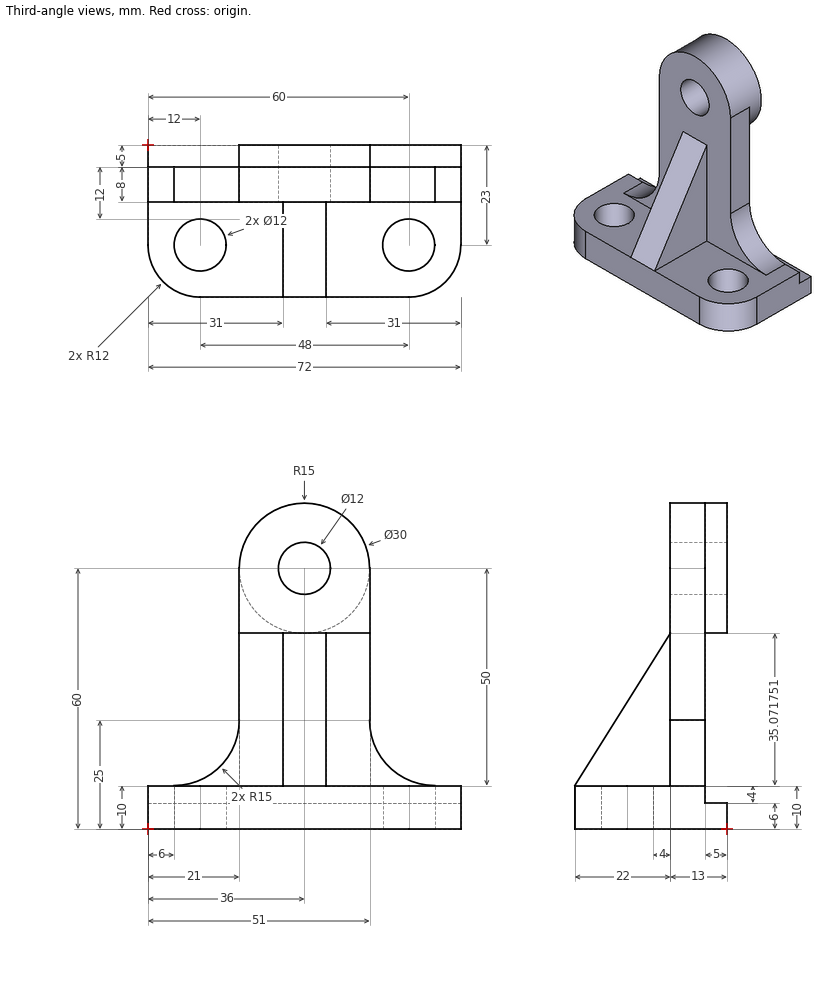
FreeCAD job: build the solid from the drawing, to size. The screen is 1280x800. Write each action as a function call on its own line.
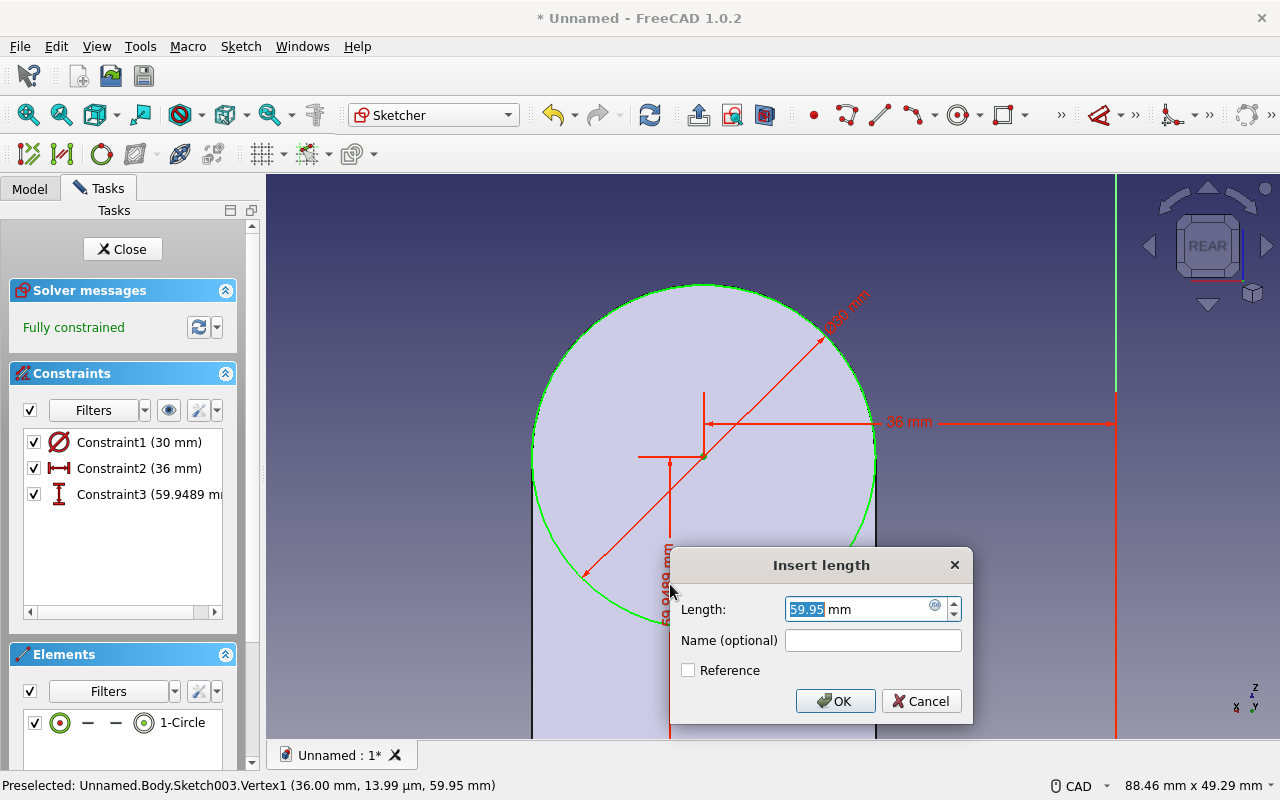
text(60)
key(Return)
key(Escape)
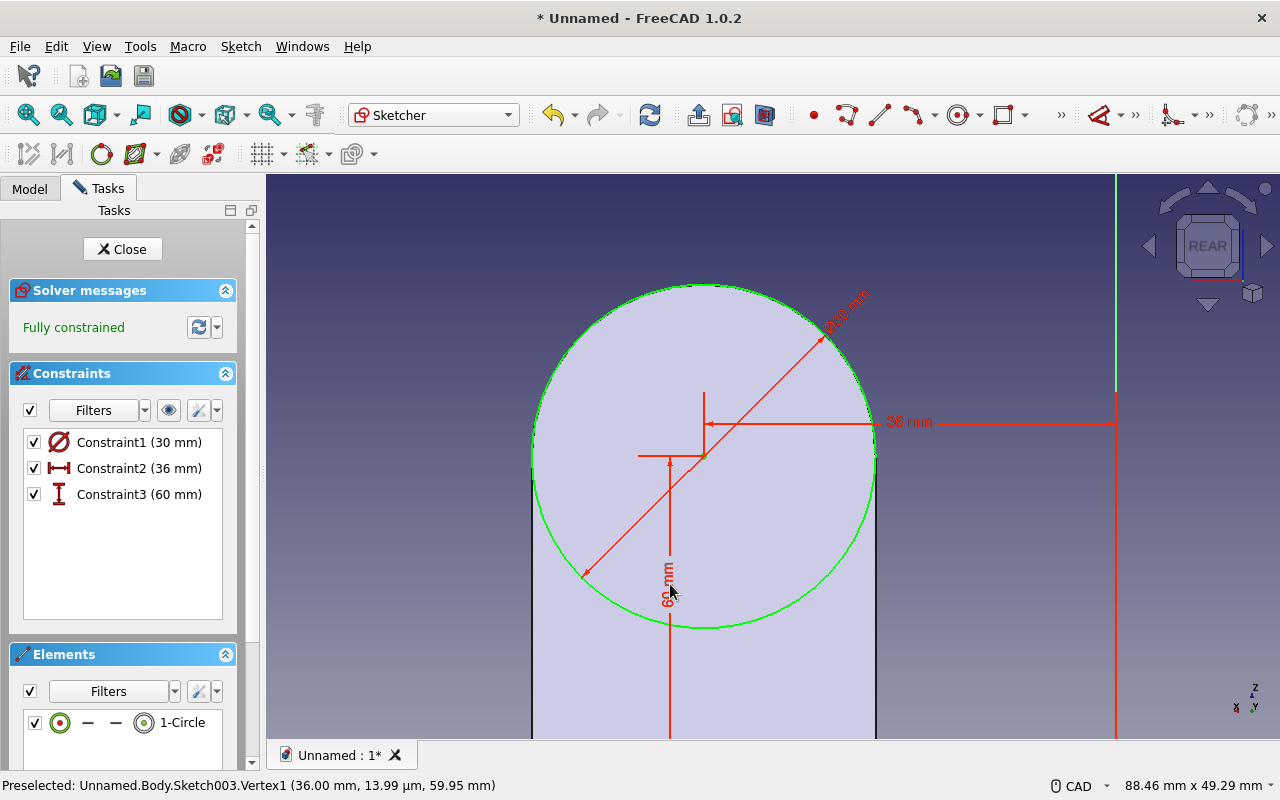
click(123, 249)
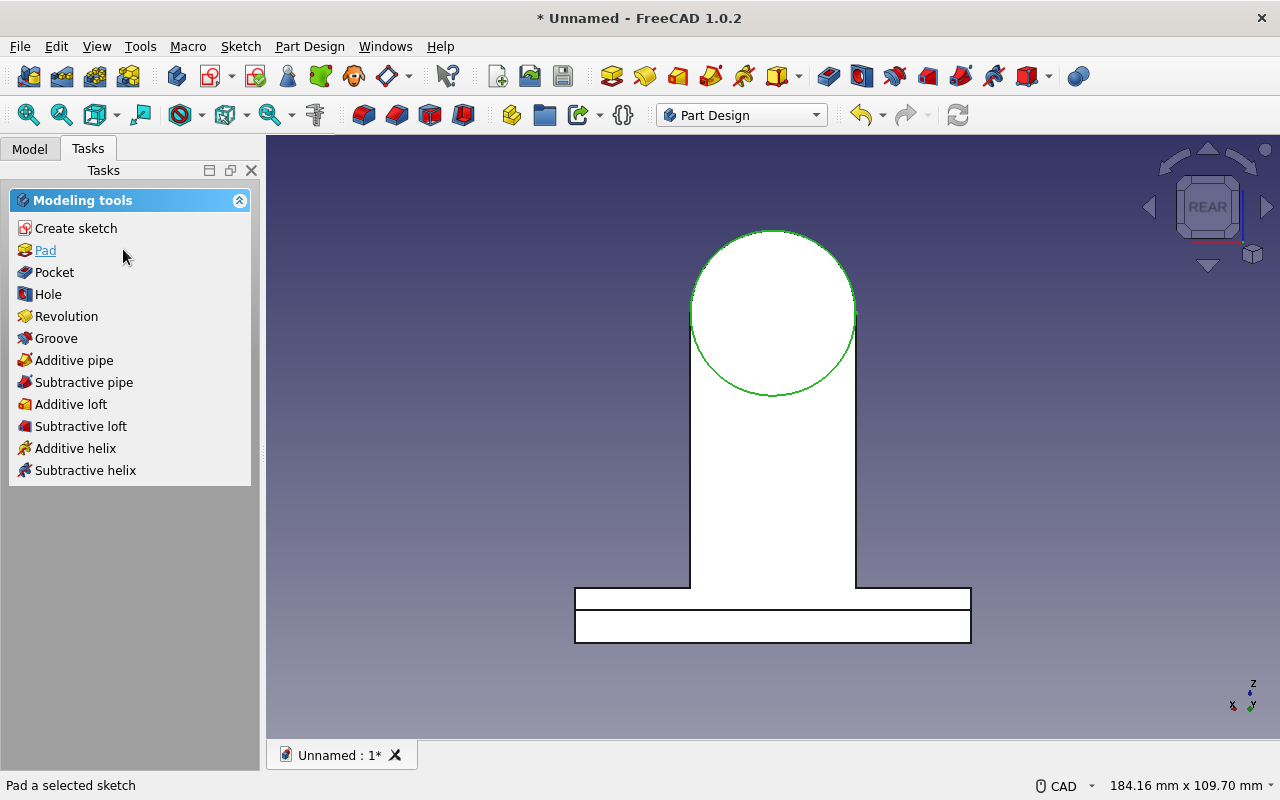
click(612, 76)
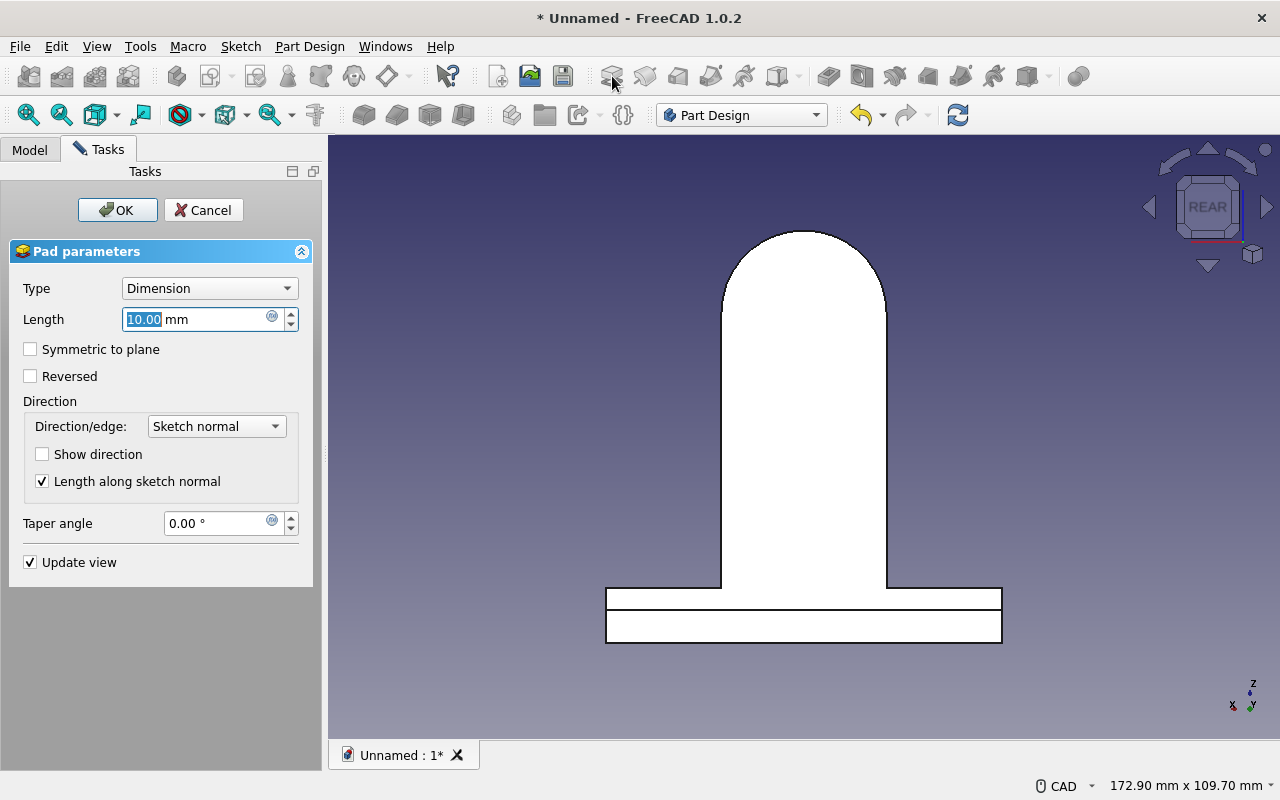
text(5)
key(Tab)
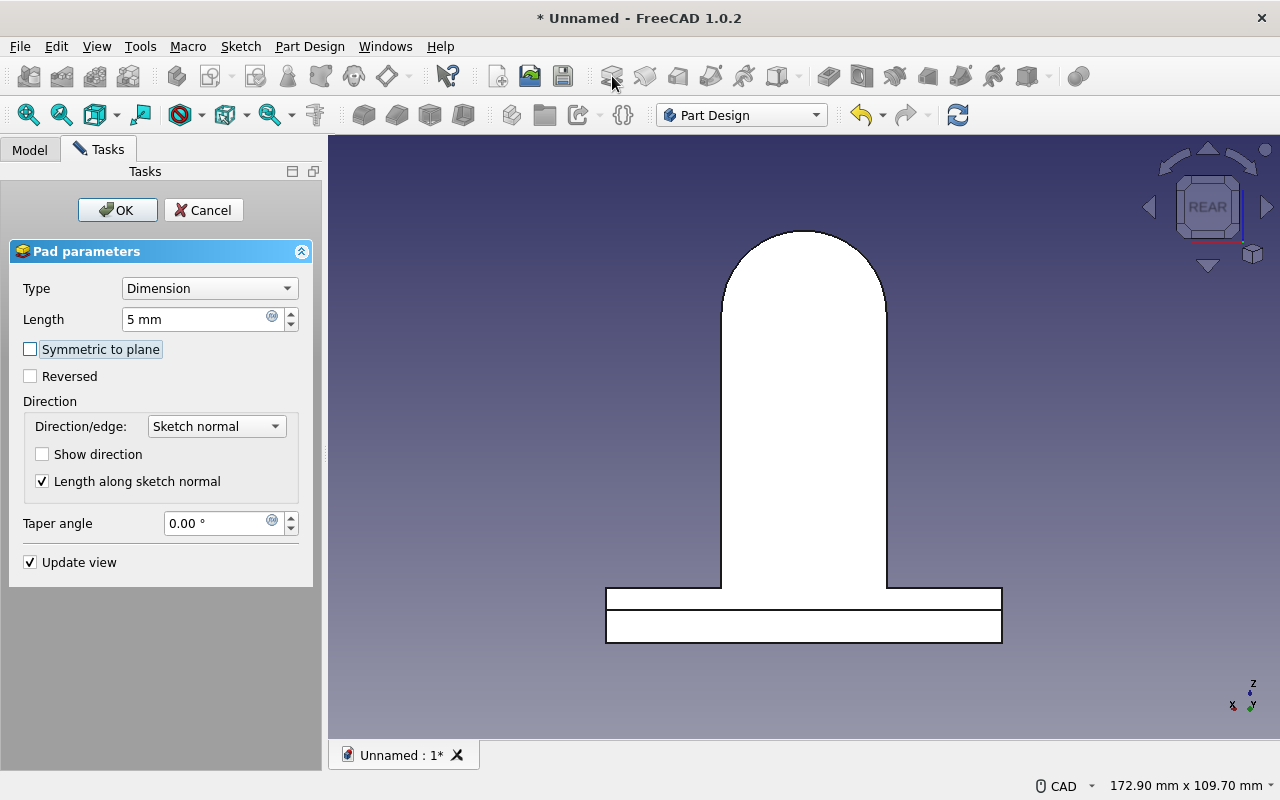
click(31, 376)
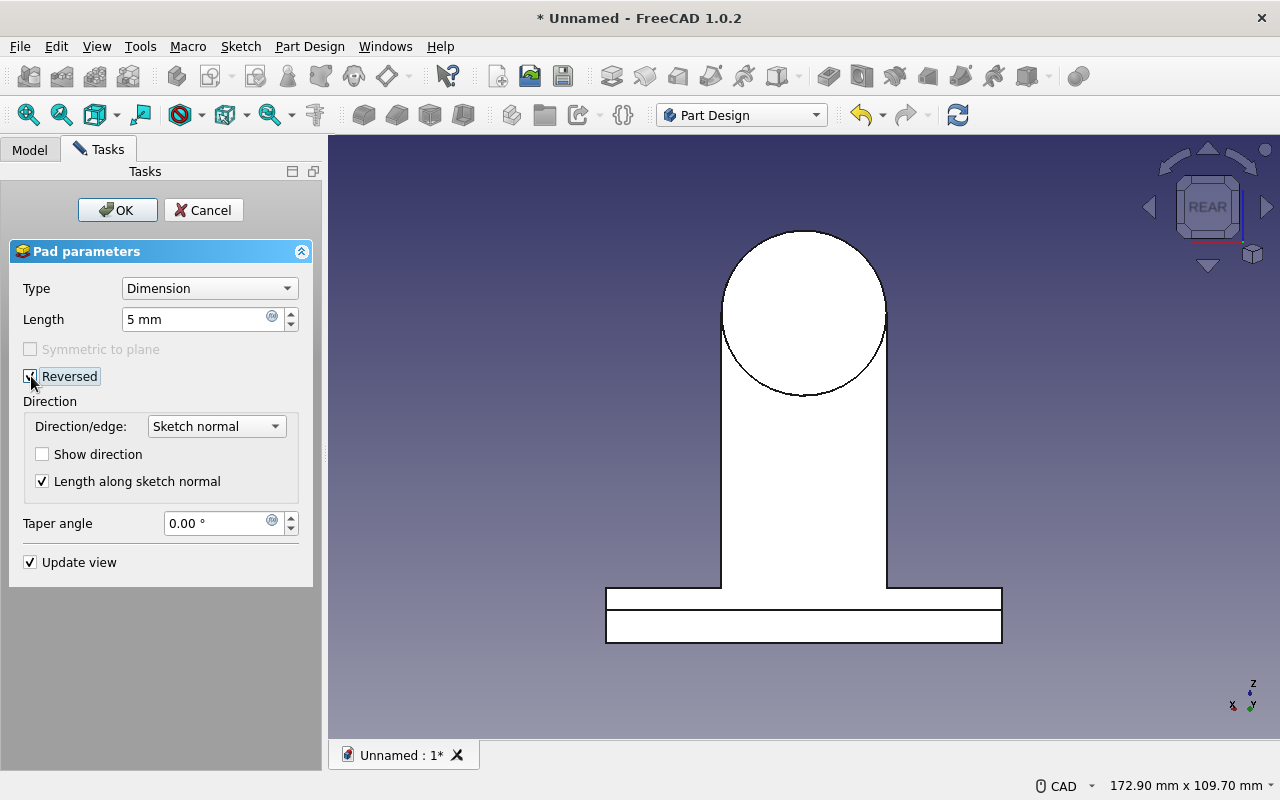
click(118, 210)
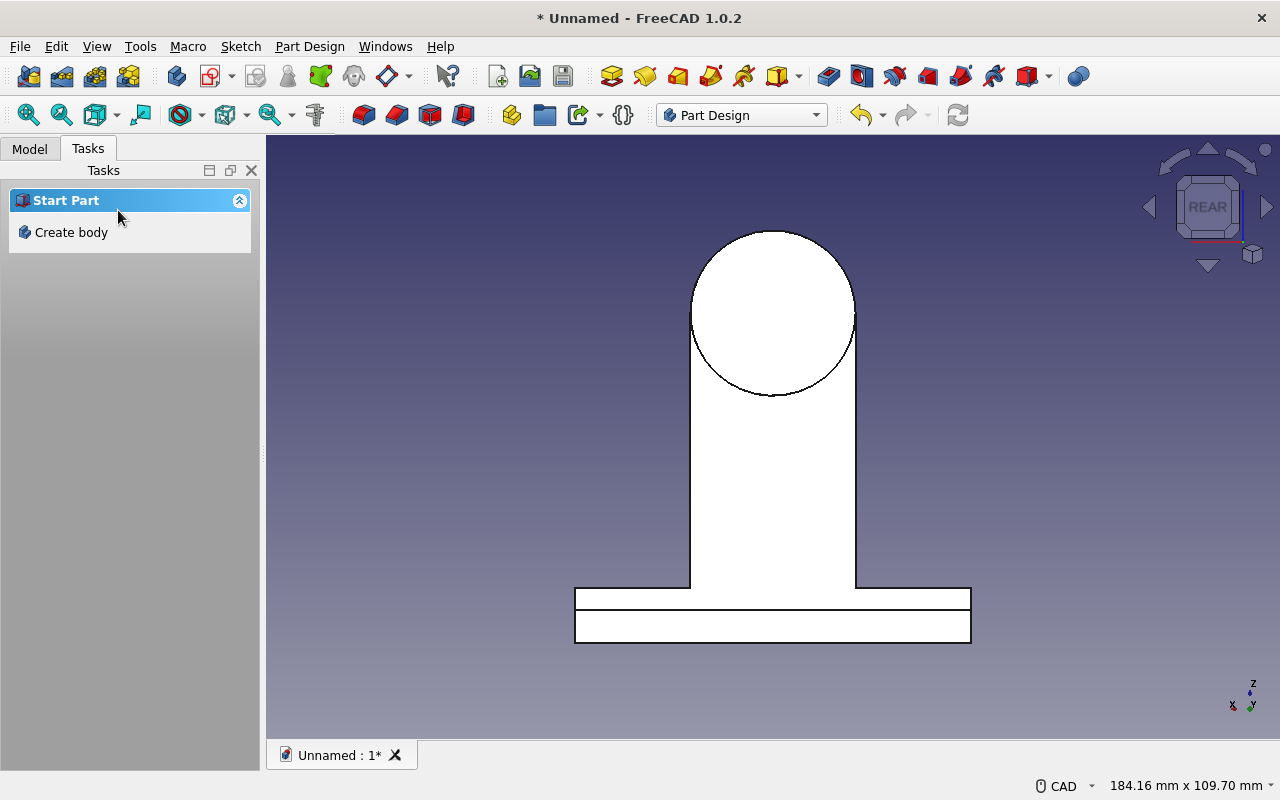
click(30, 148)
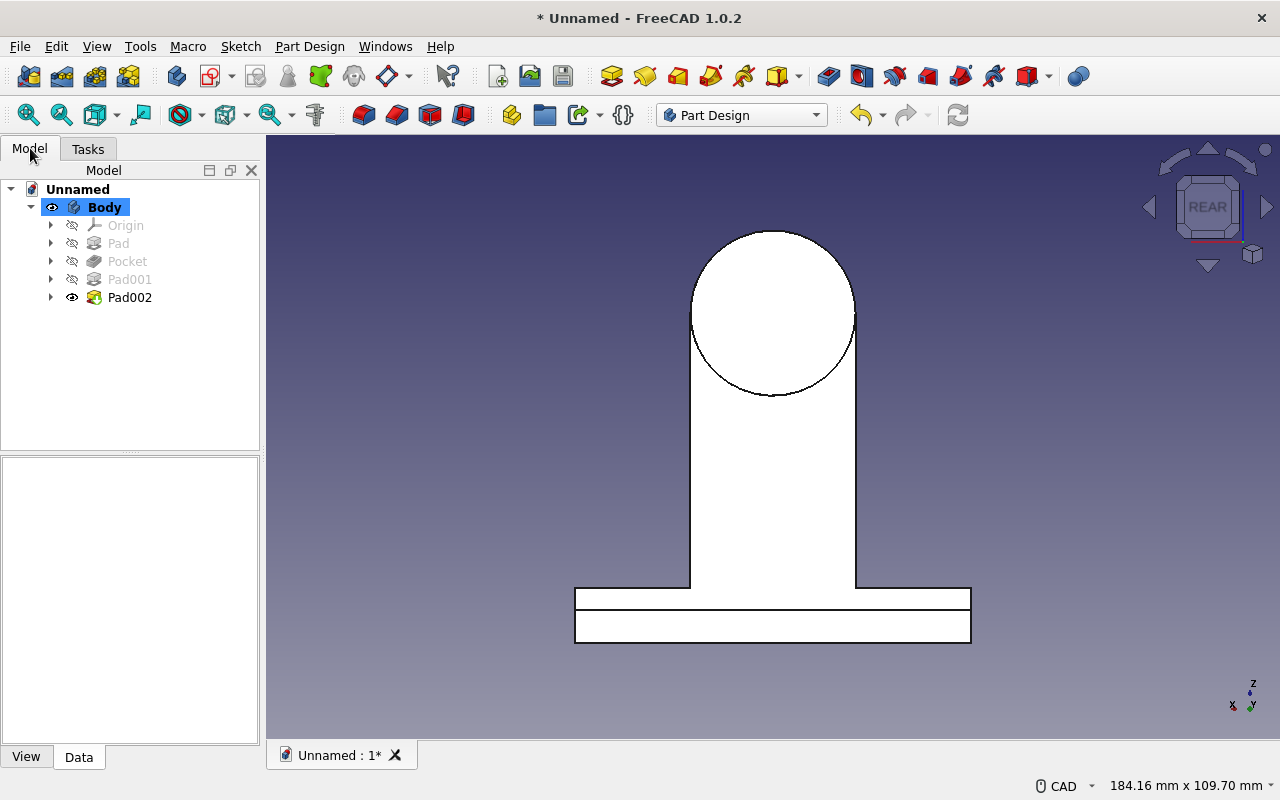
click(51, 225)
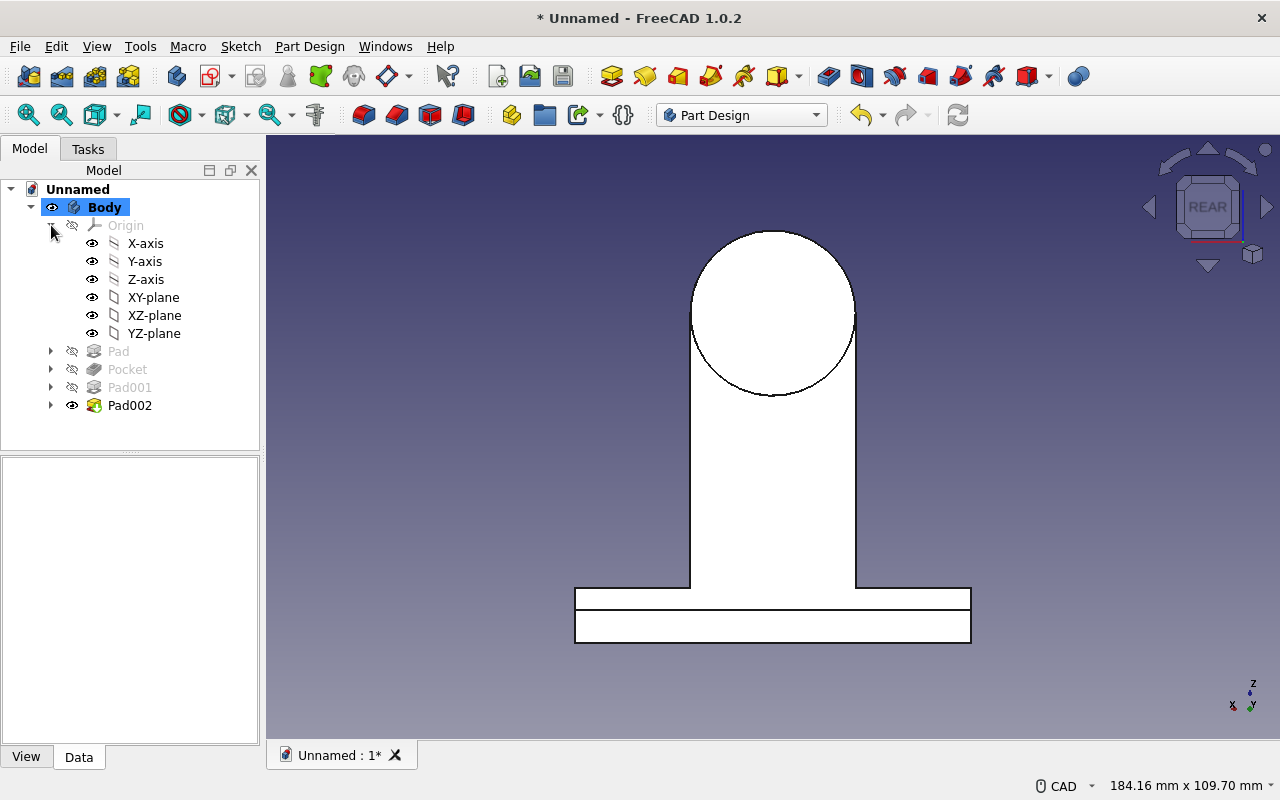
click(137, 315)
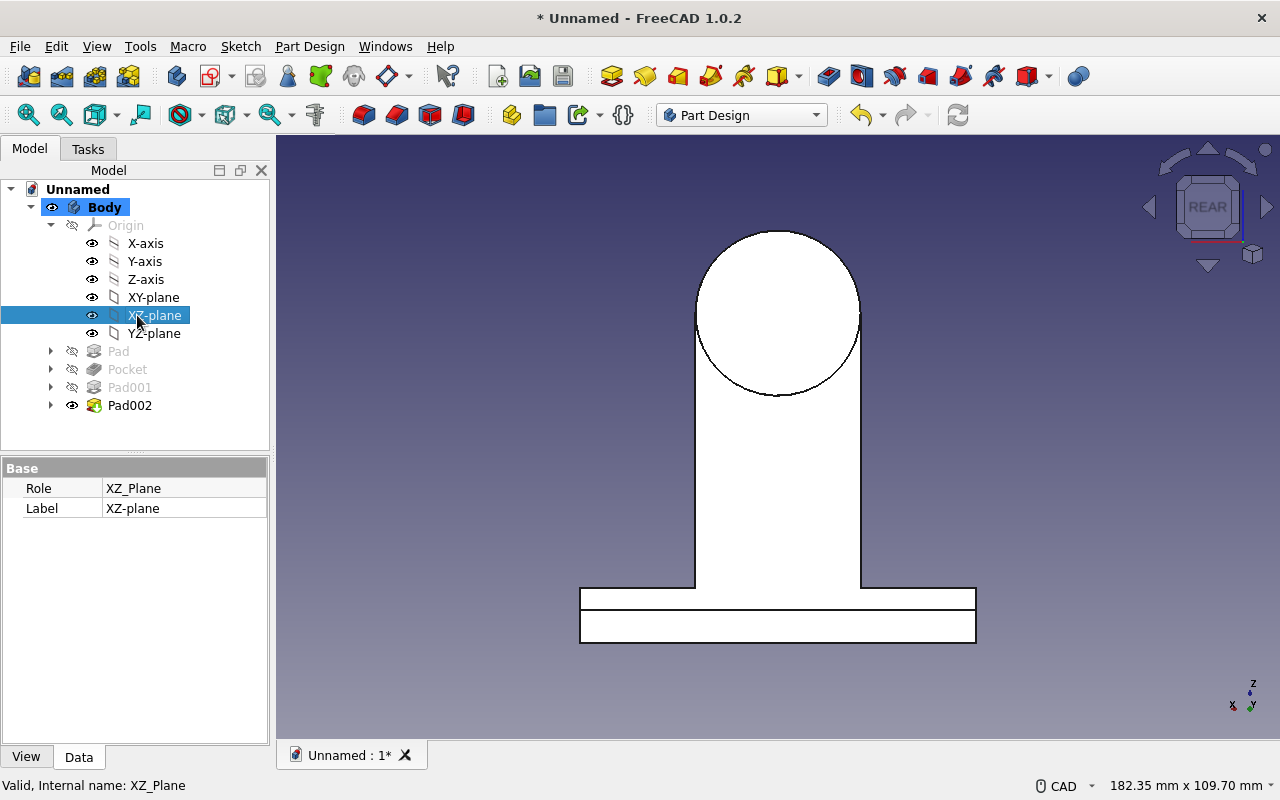
click(386, 76)